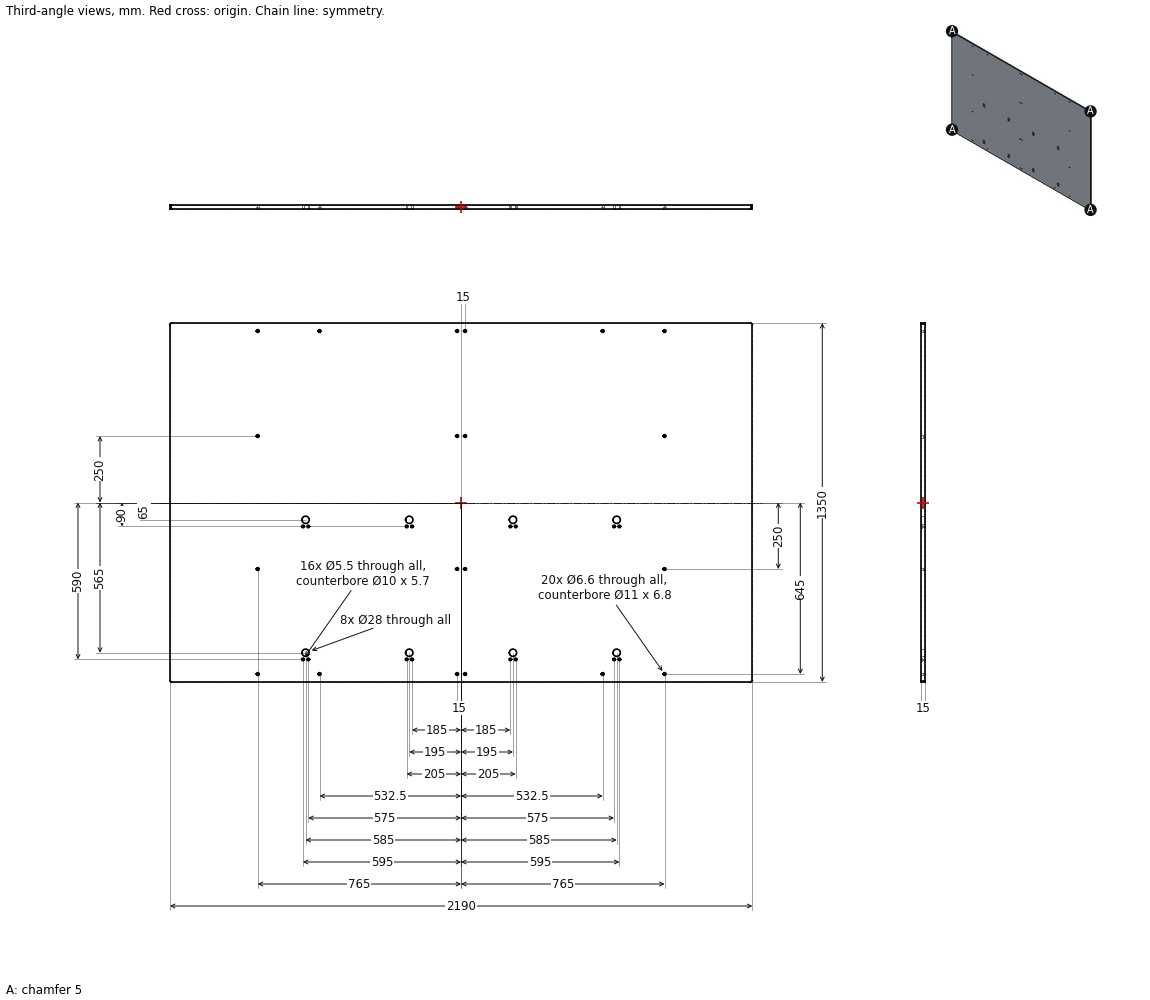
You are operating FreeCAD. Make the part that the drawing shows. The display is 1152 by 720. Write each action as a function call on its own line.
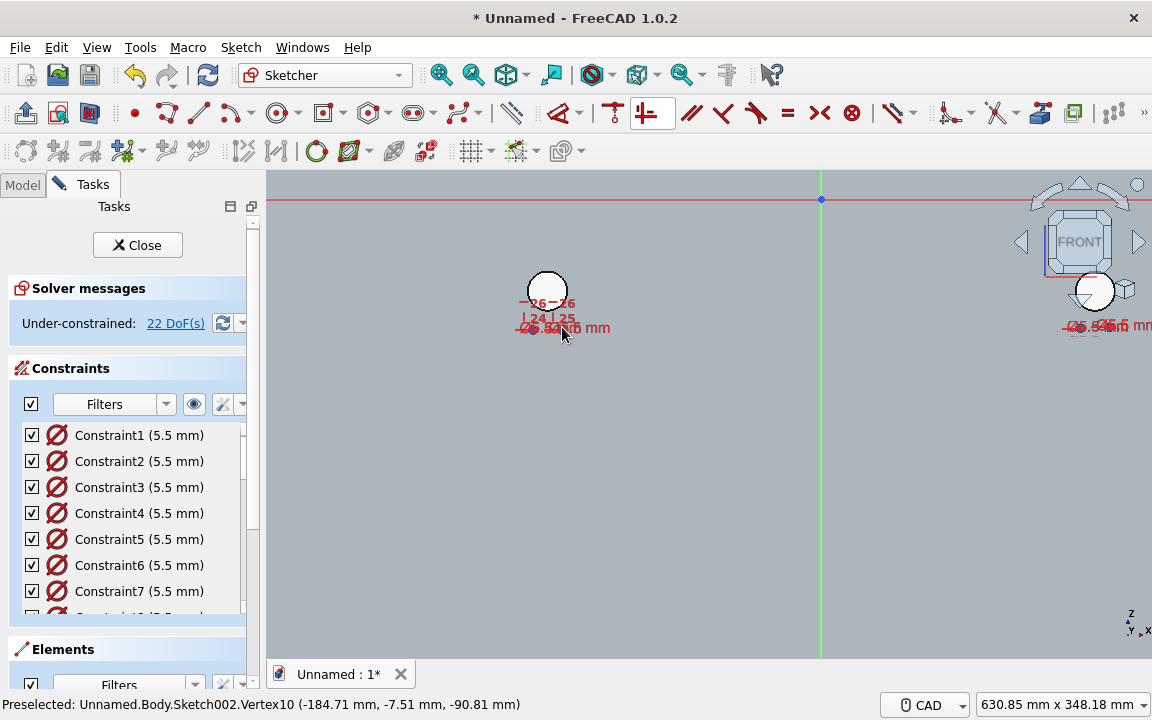
scroll(563, 328, down, 6)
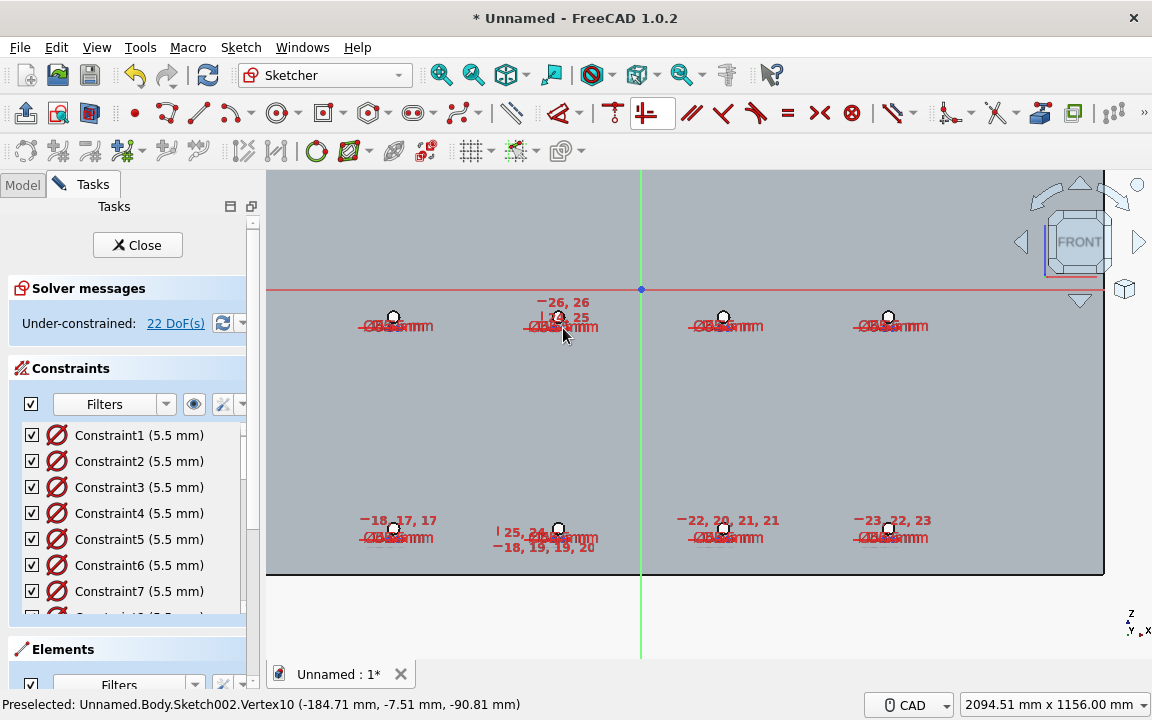
scroll(719, 540, up, 2)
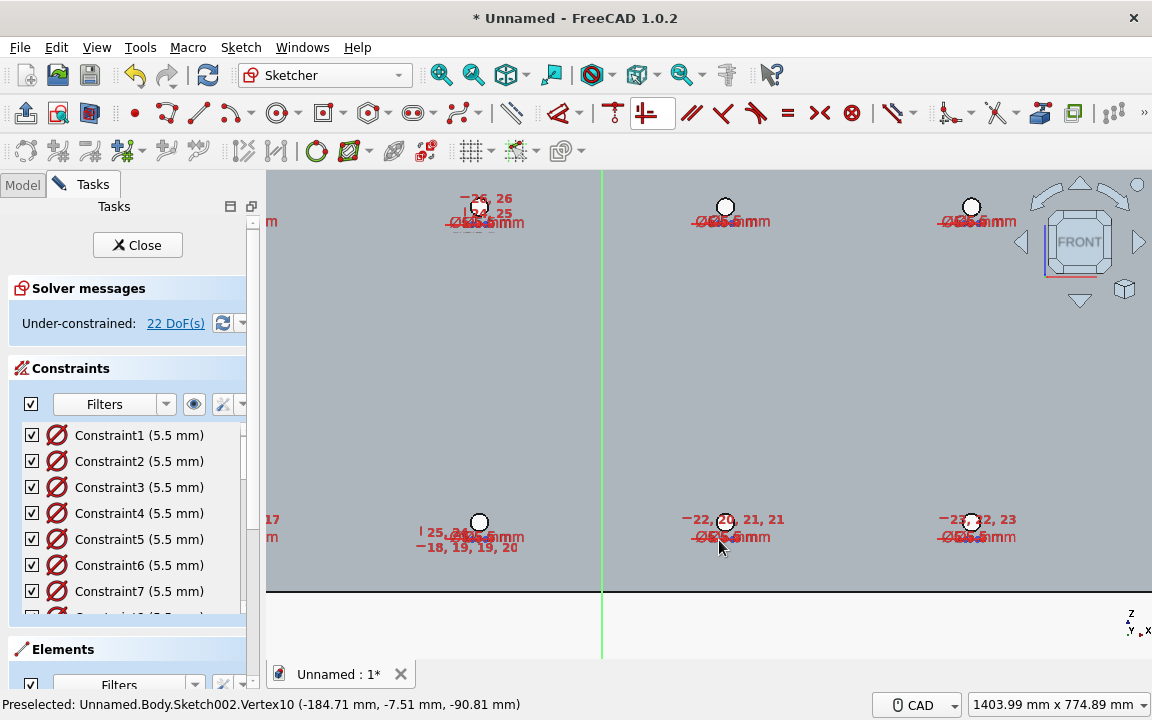
click(719, 539)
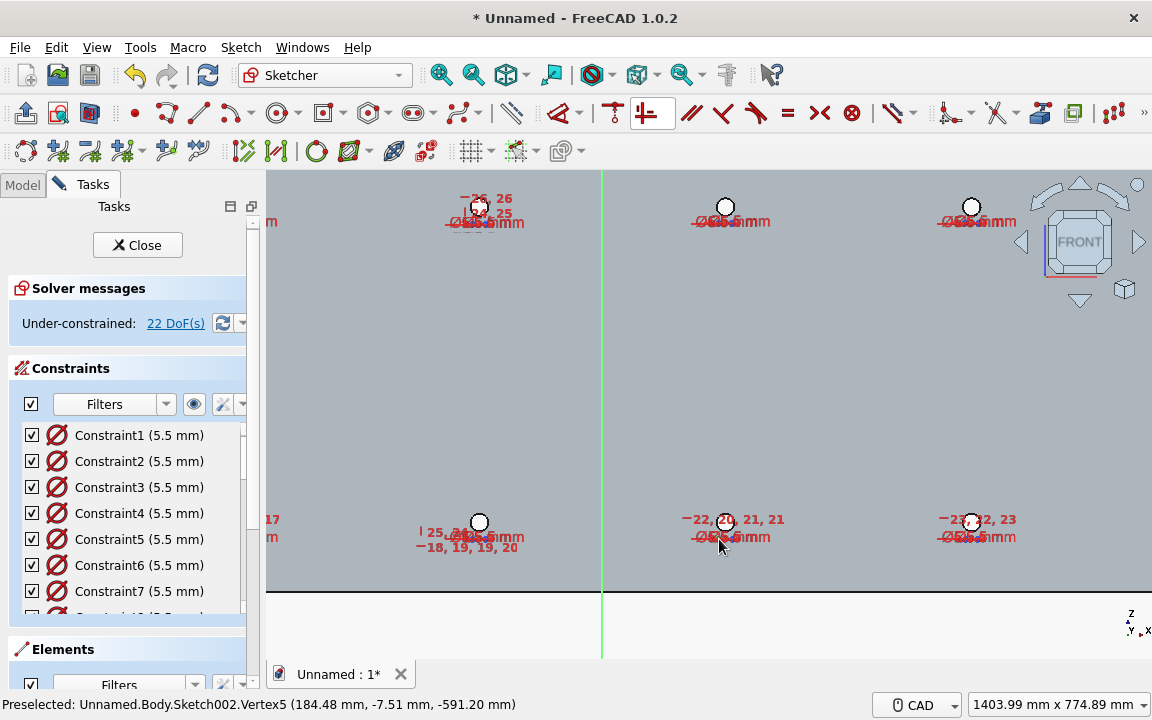
click(719, 224)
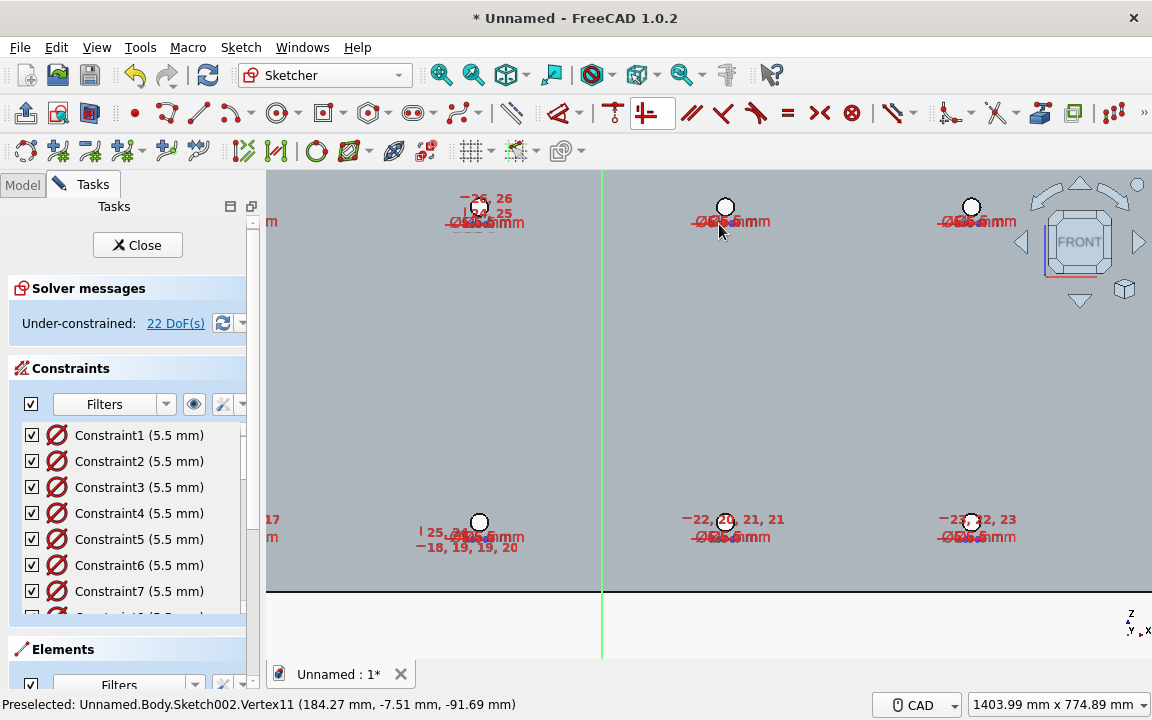
key(v)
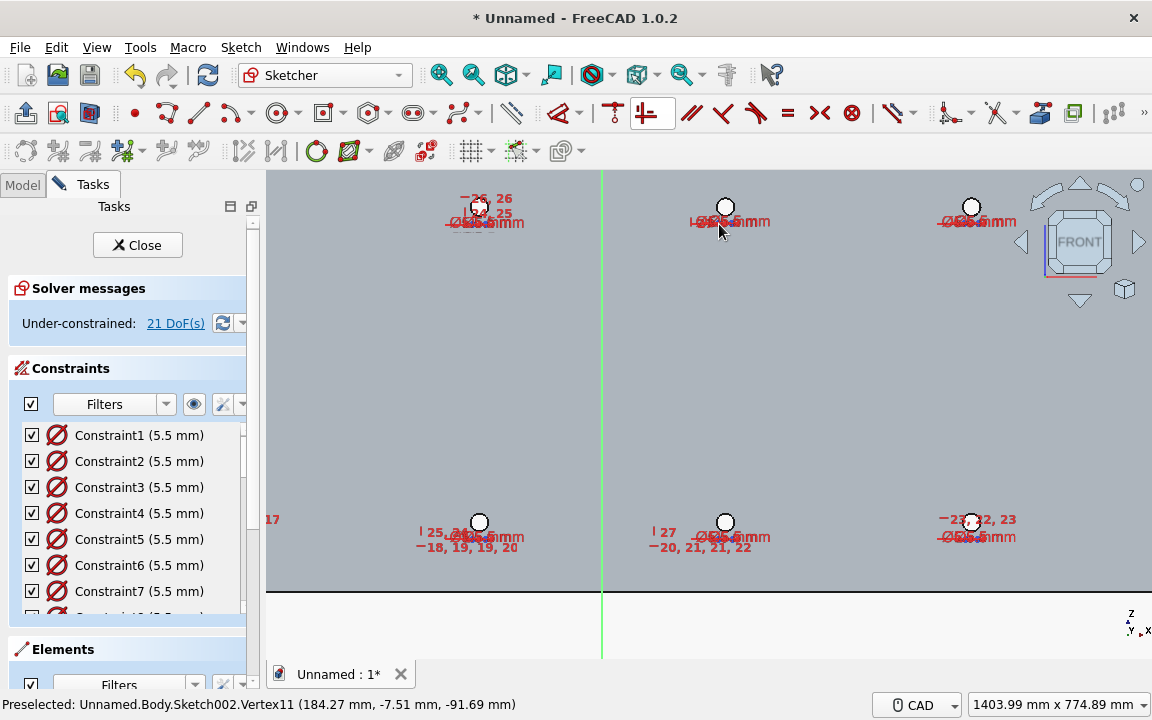
click(486, 225)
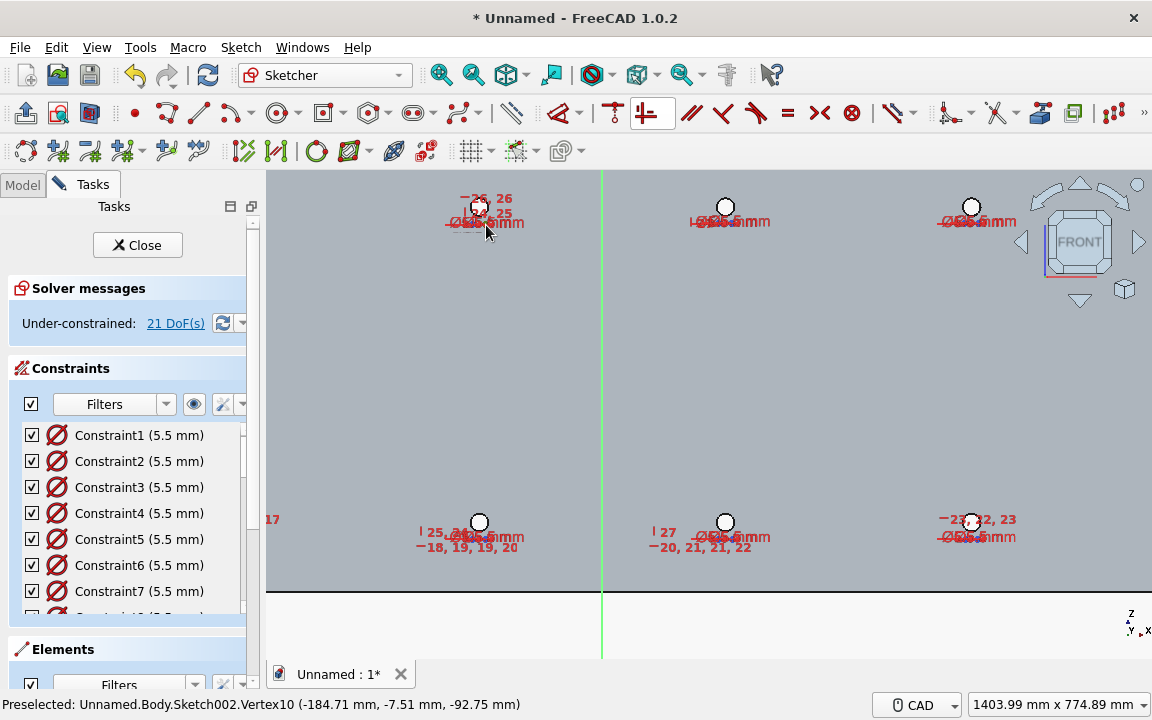
click(719, 224)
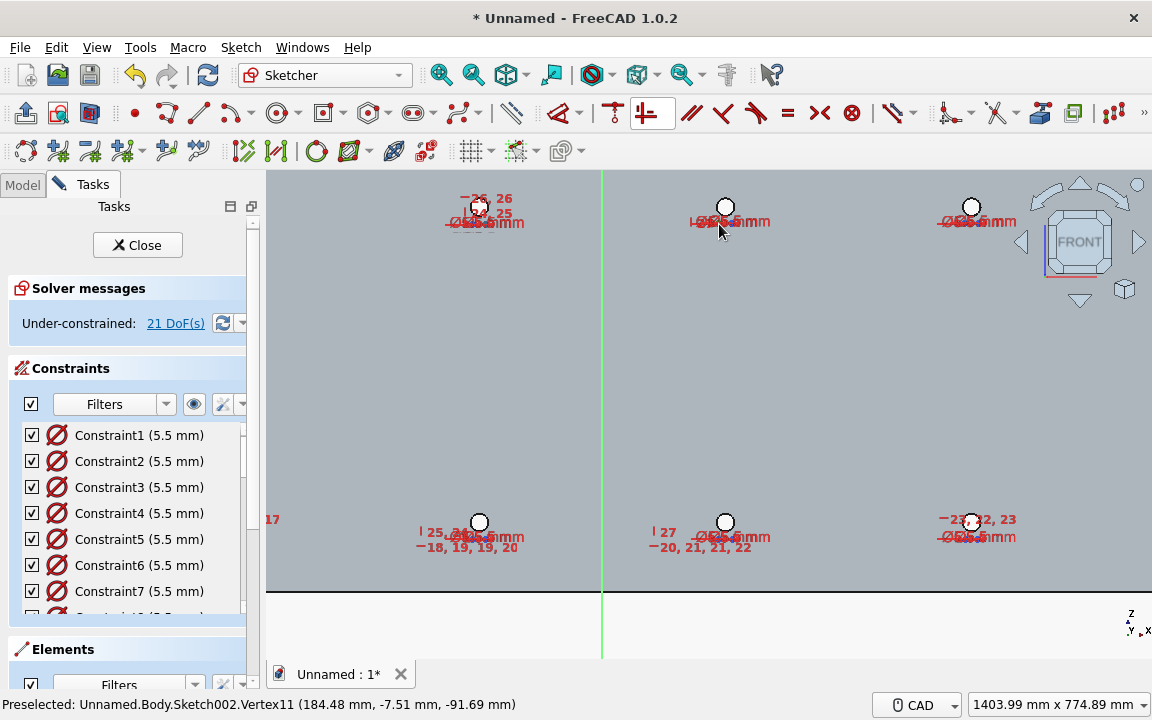
key(h)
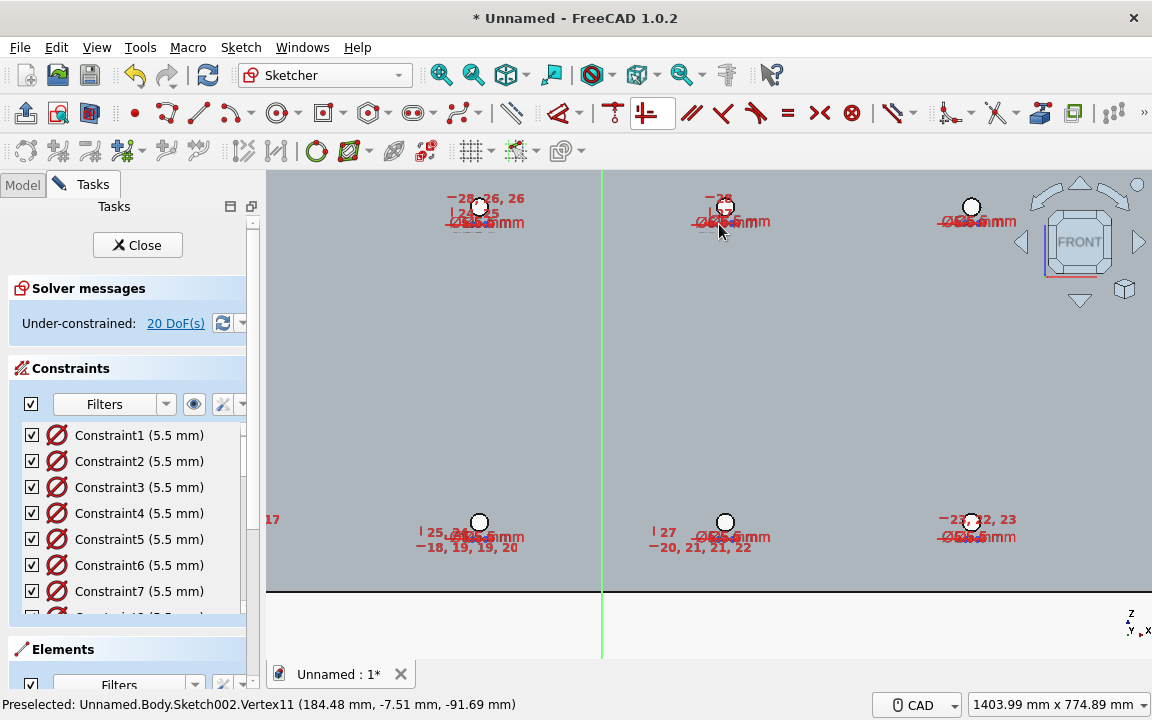
click(732, 539)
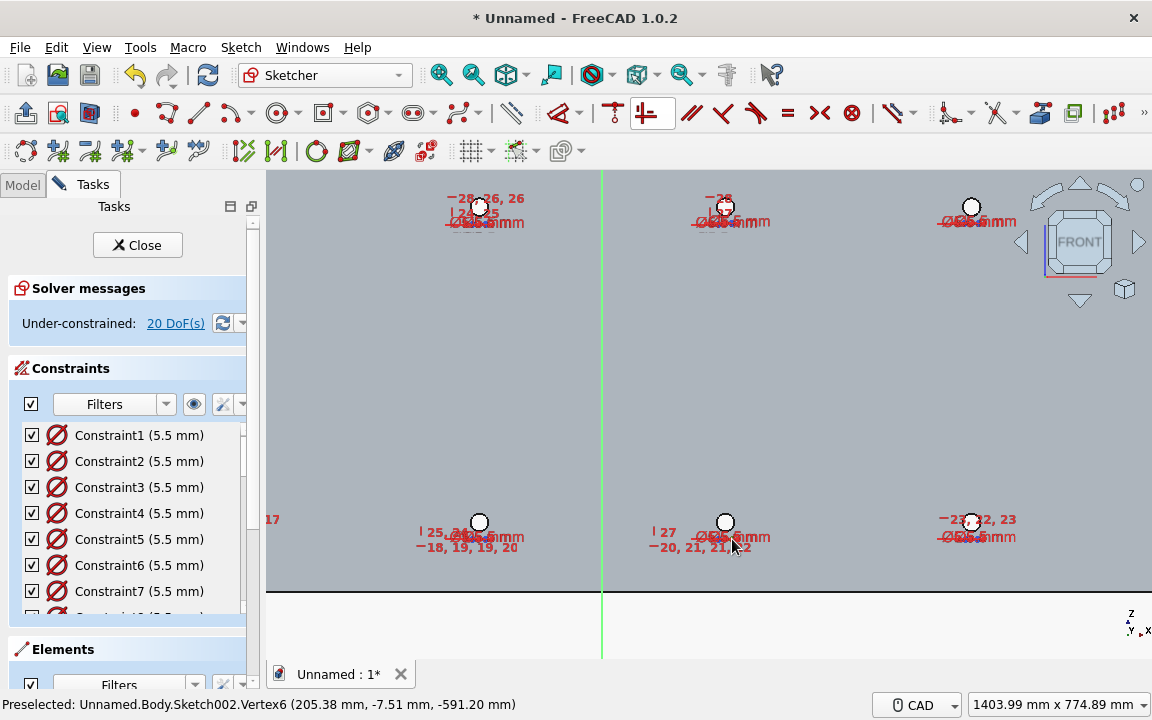
click(732, 223)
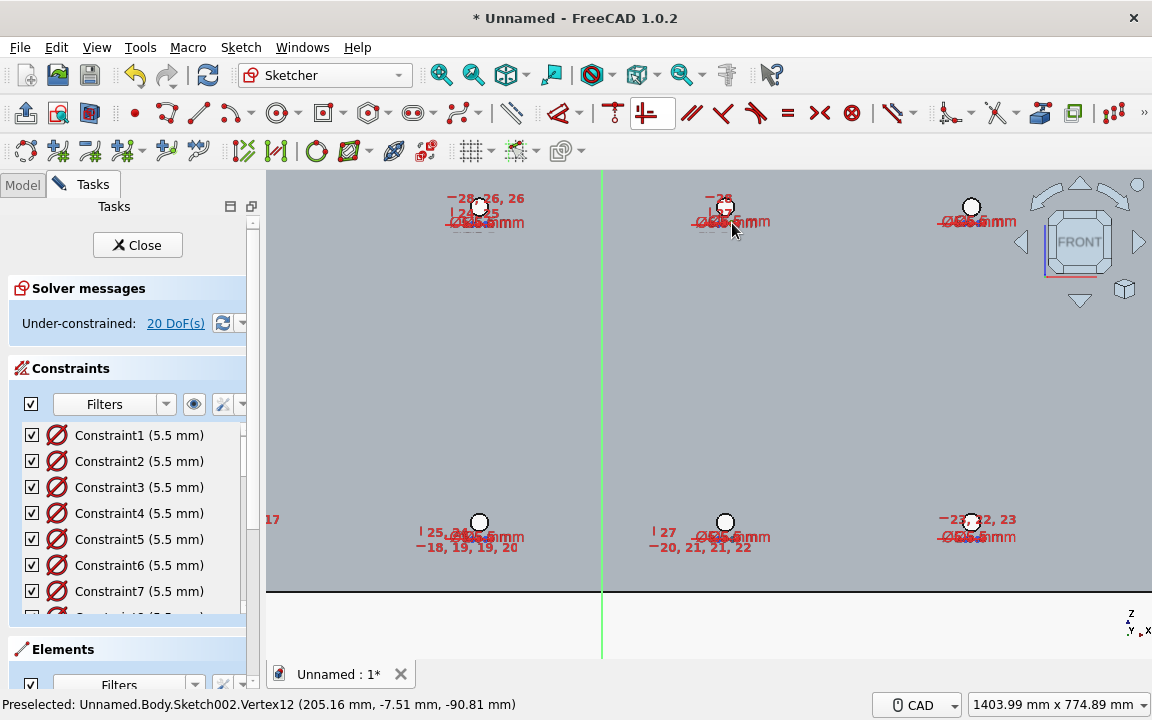
click(670, 114)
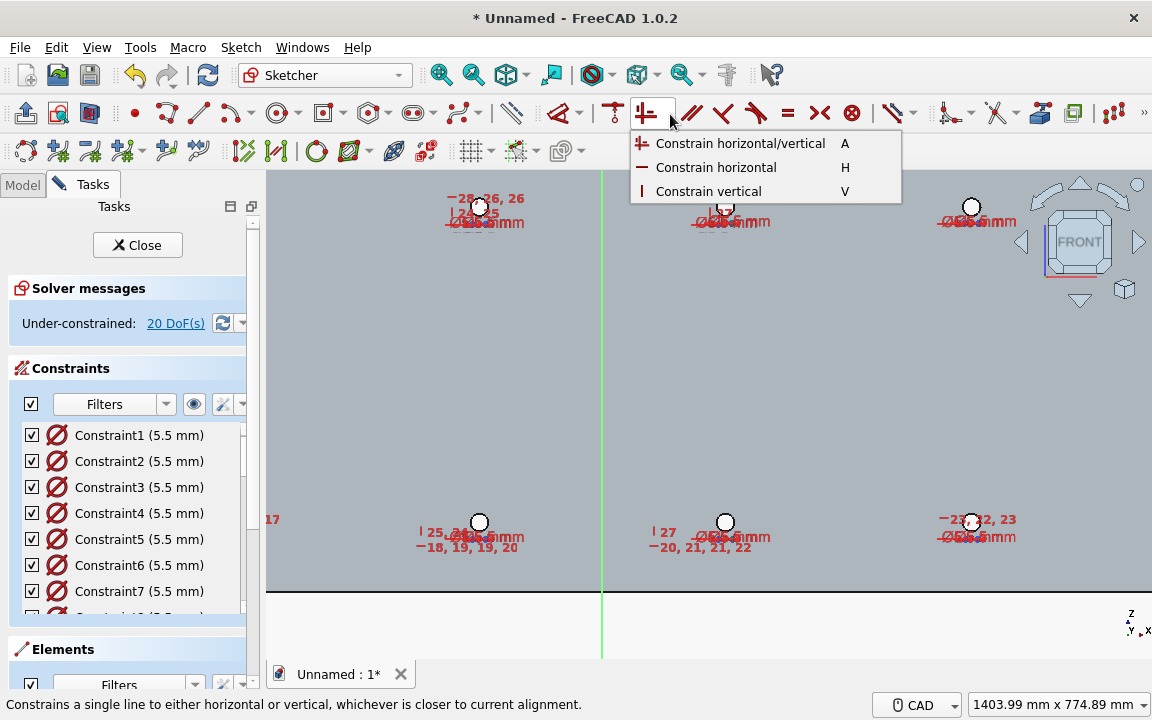
click(766, 191)